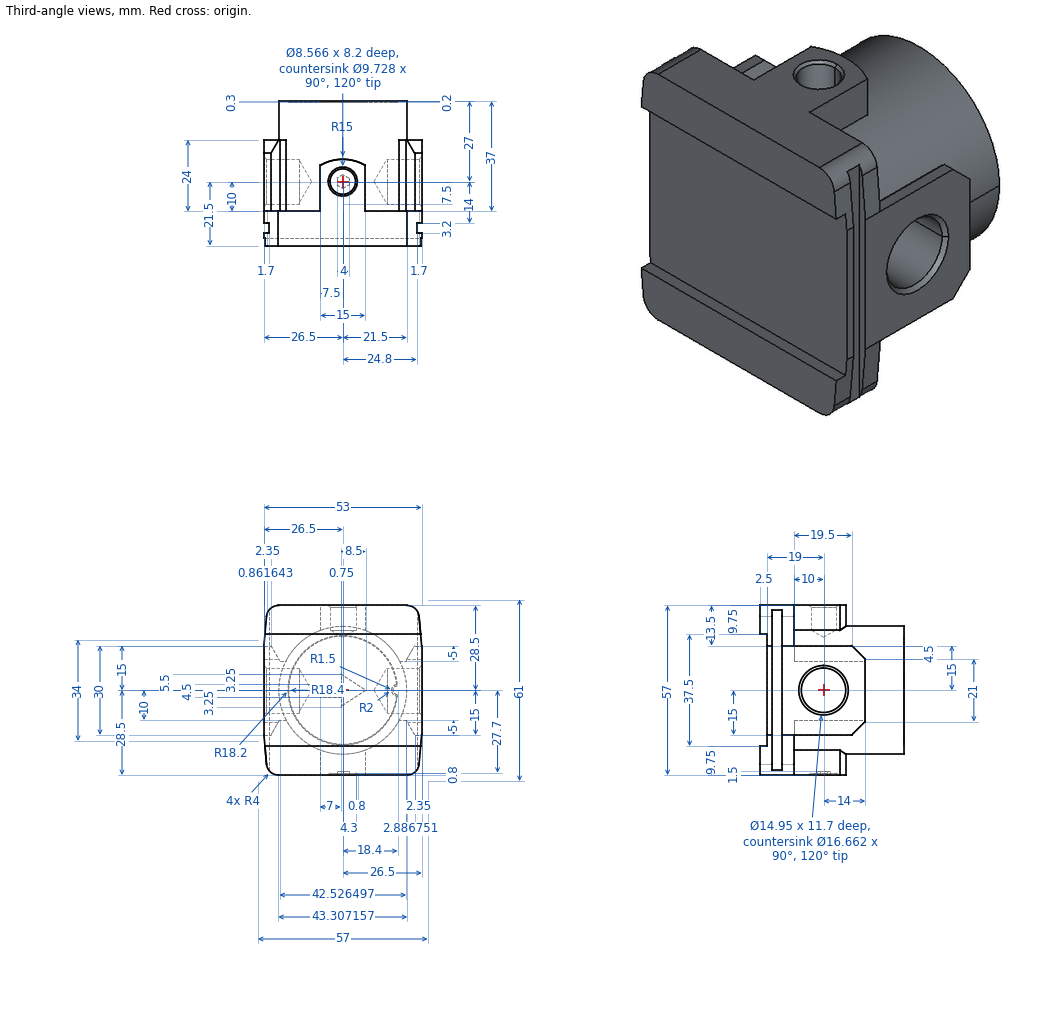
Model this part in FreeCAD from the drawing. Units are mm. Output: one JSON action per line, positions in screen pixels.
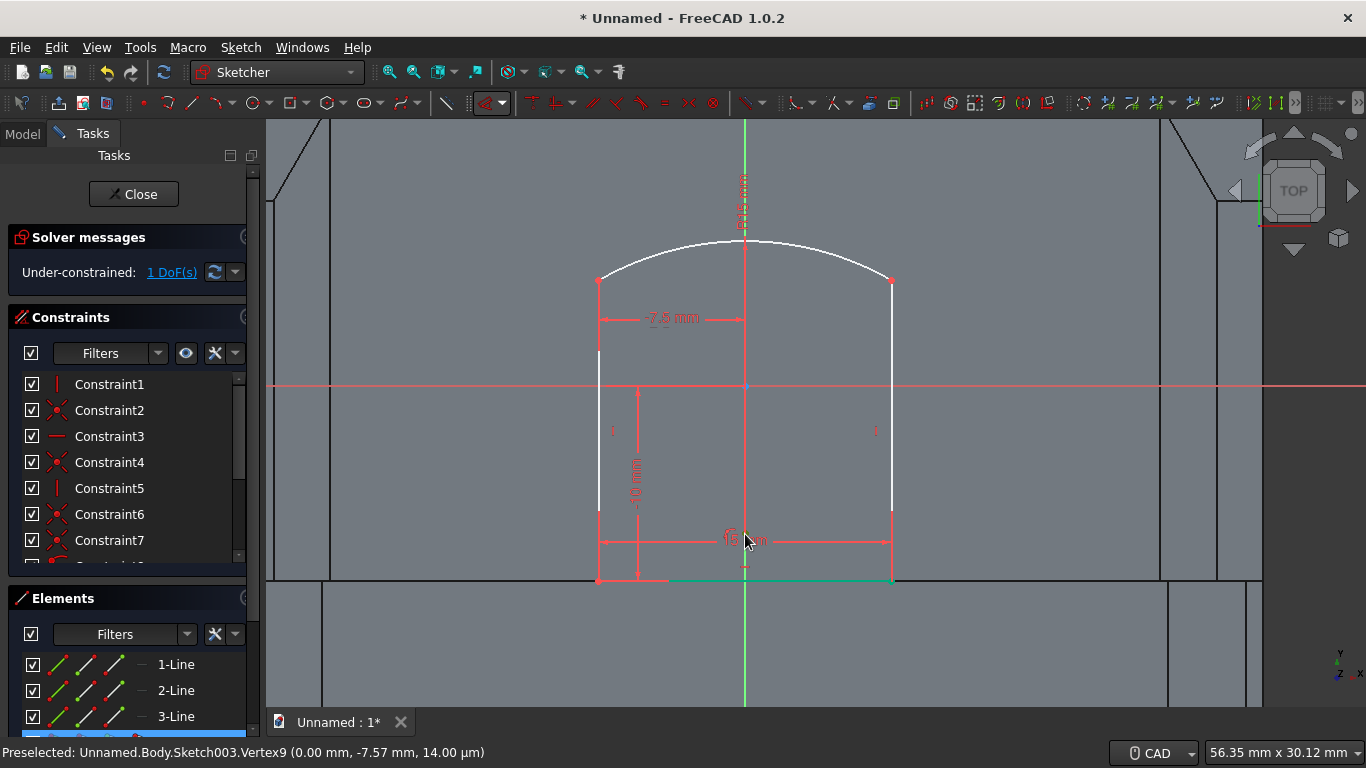
{"action": "key", "text": "i"}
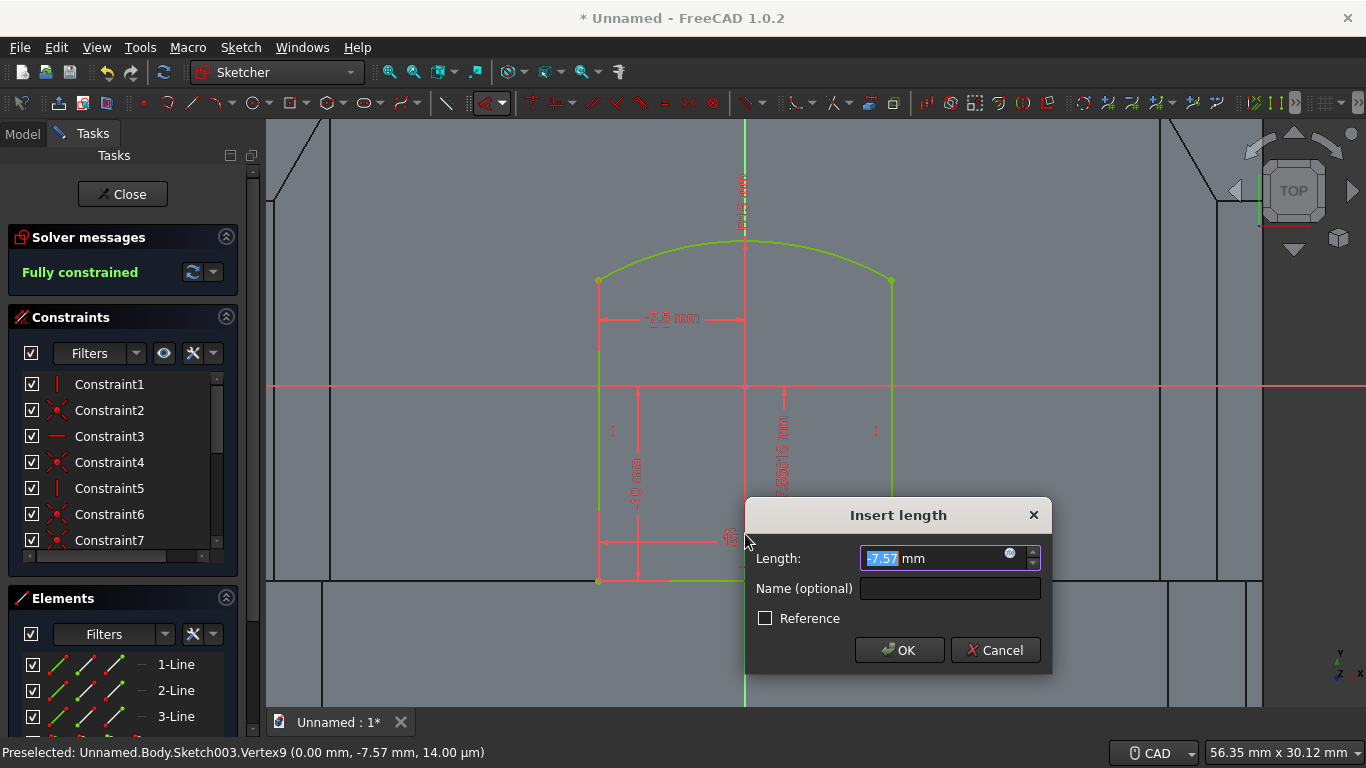
{"action": "type", "text": "-7.5"}
{"action": "key", "text": "Return"}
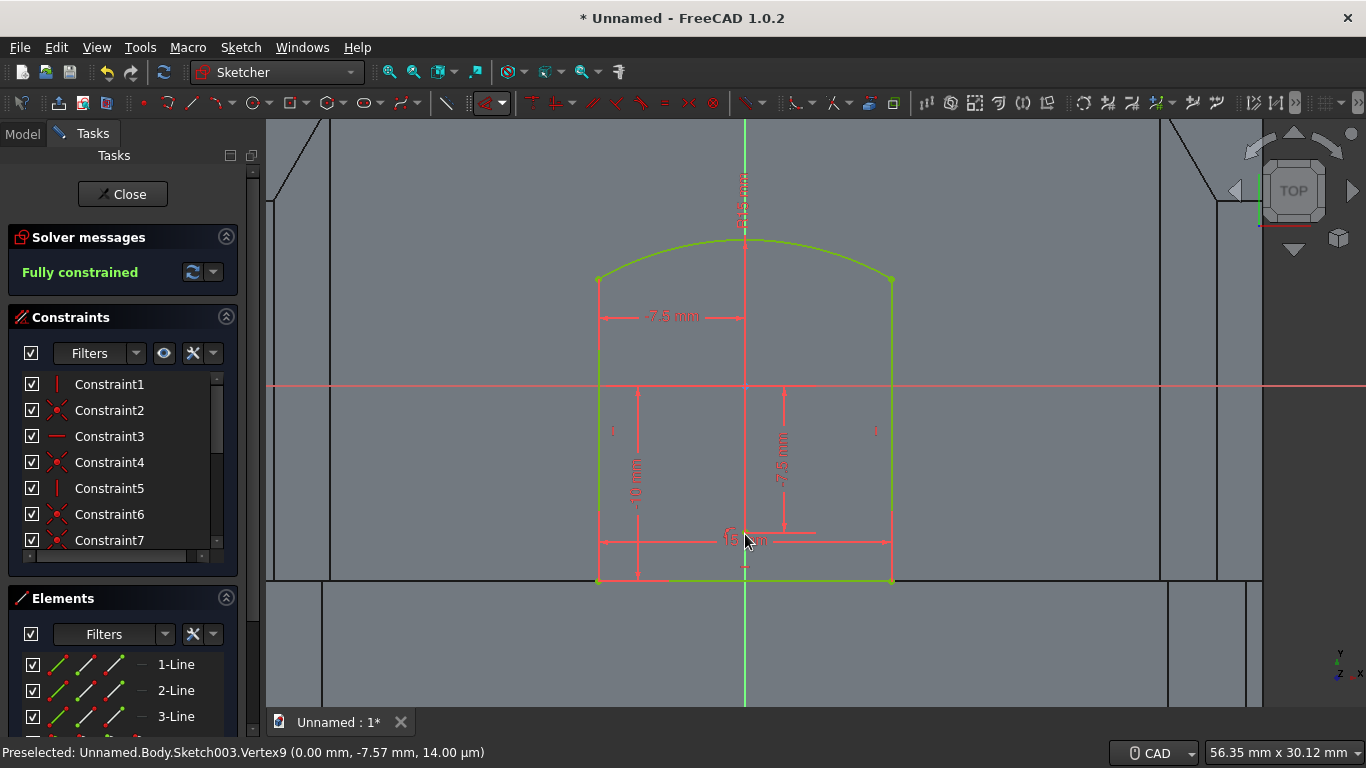
{"action": "left_click", "coordinate": [123, 194]}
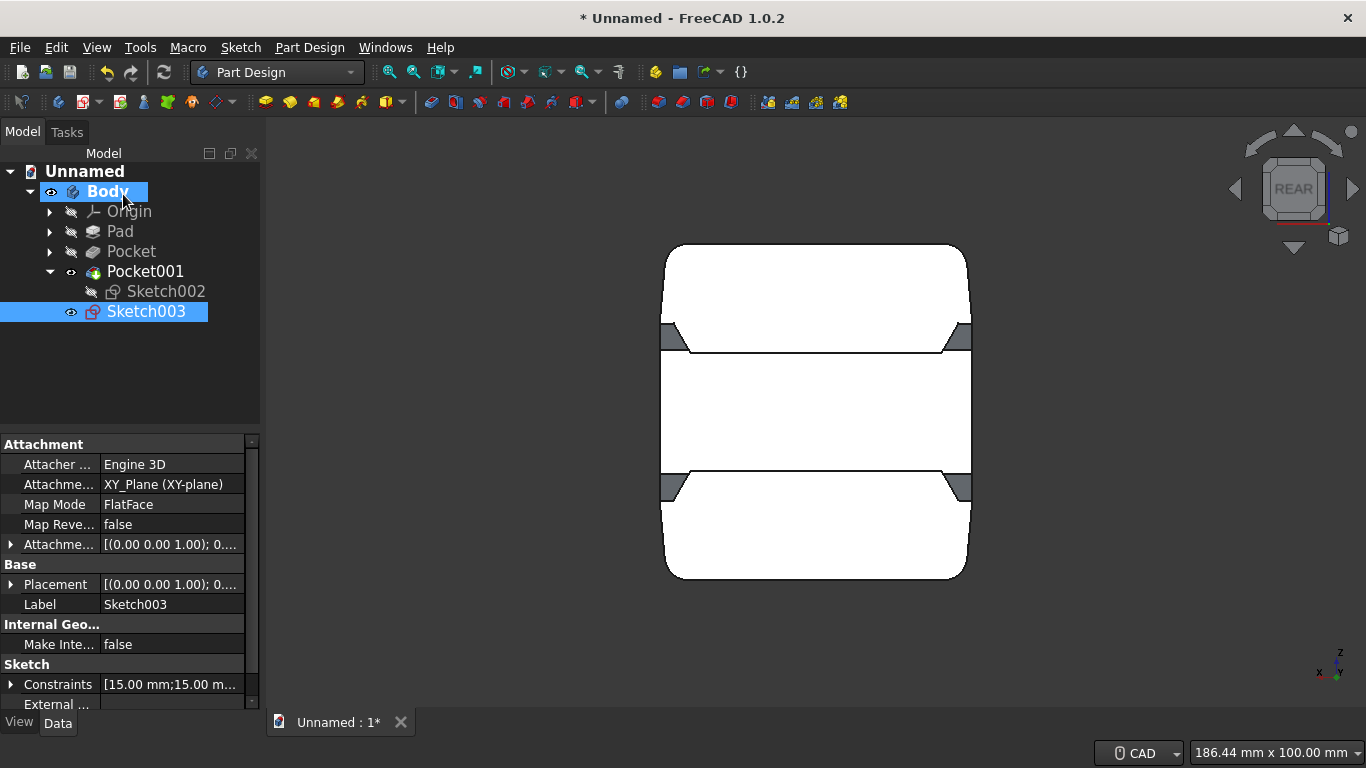
{"action": "left_click", "coordinate": [266, 102]}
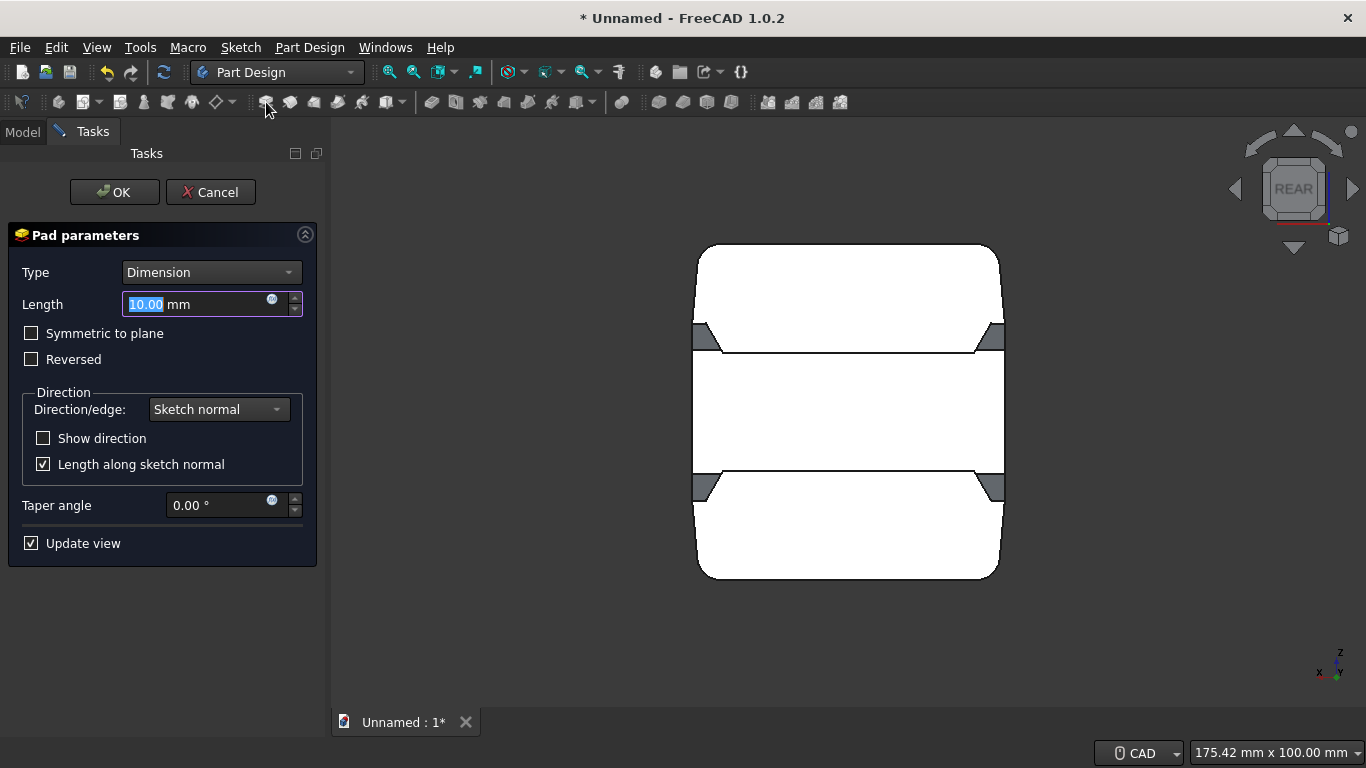
{"action": "type", "text": "57"}
{"action": "key", "text": "Tab"}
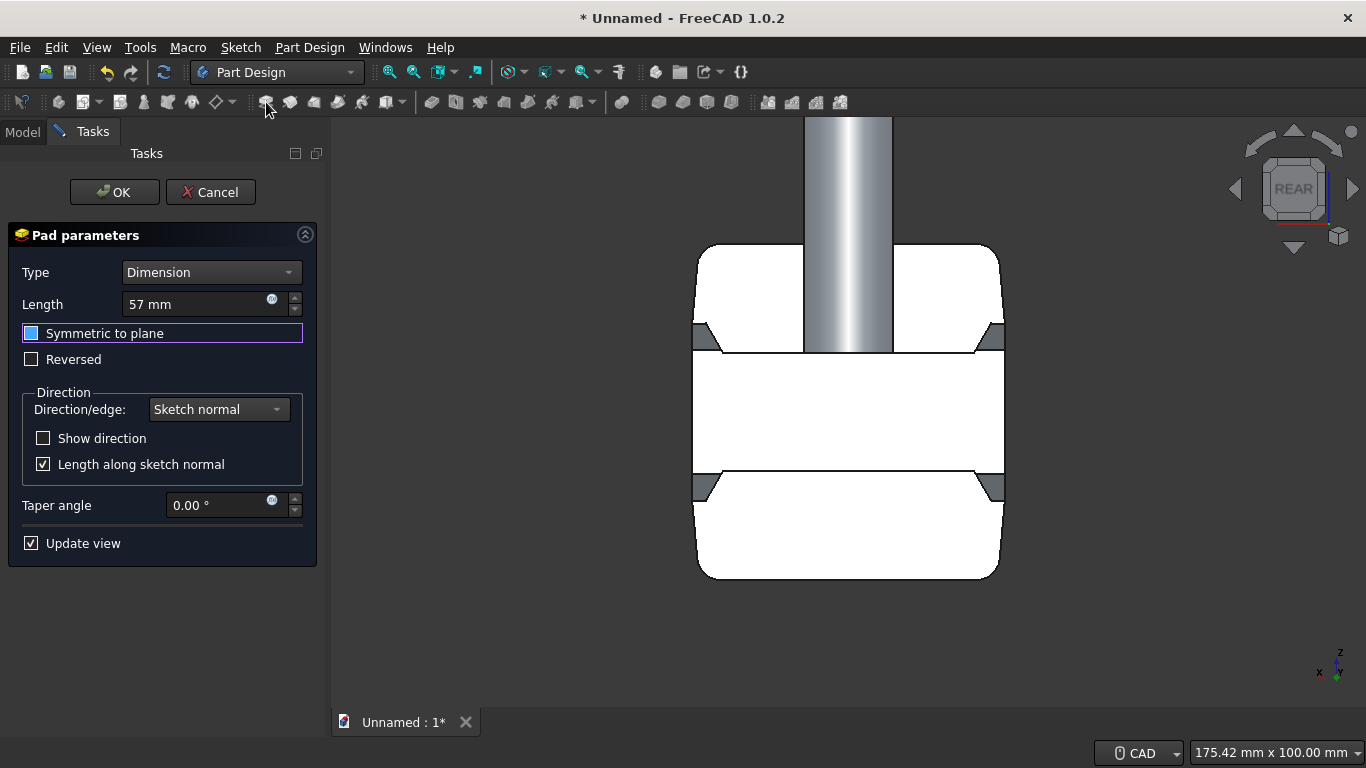
{"action": "left_click", "coordinate": [30, 333]}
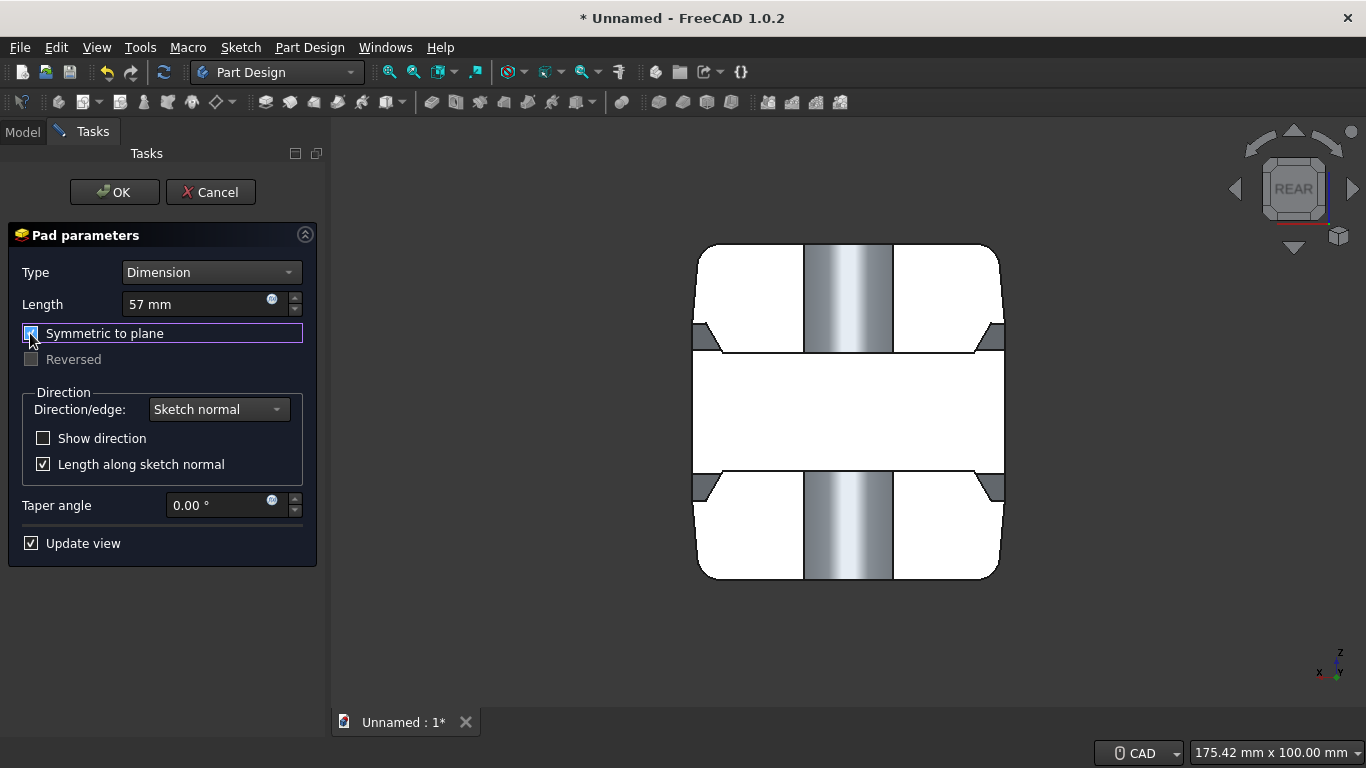
{"action": "left_click", "coordinate": [115, 192]}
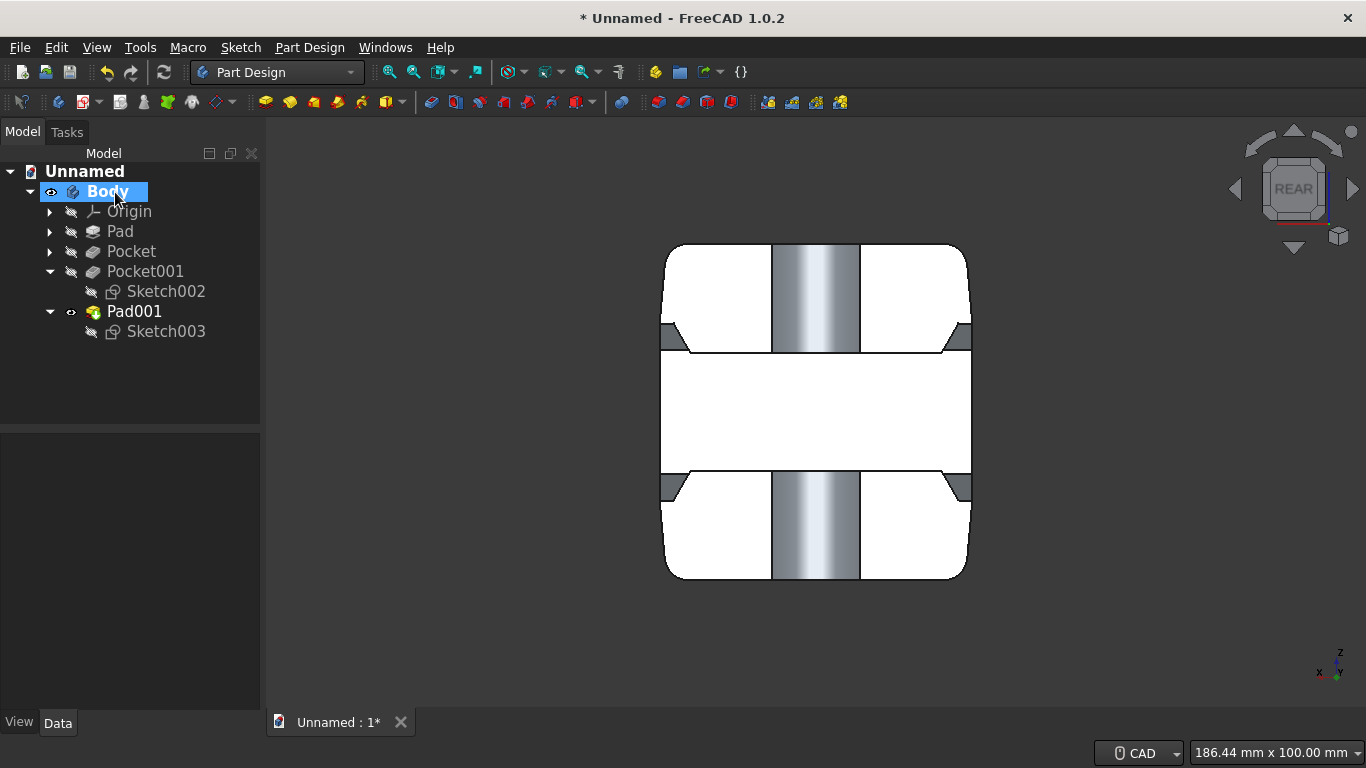
{"action": "left_click", "coordinate": [84, 102]}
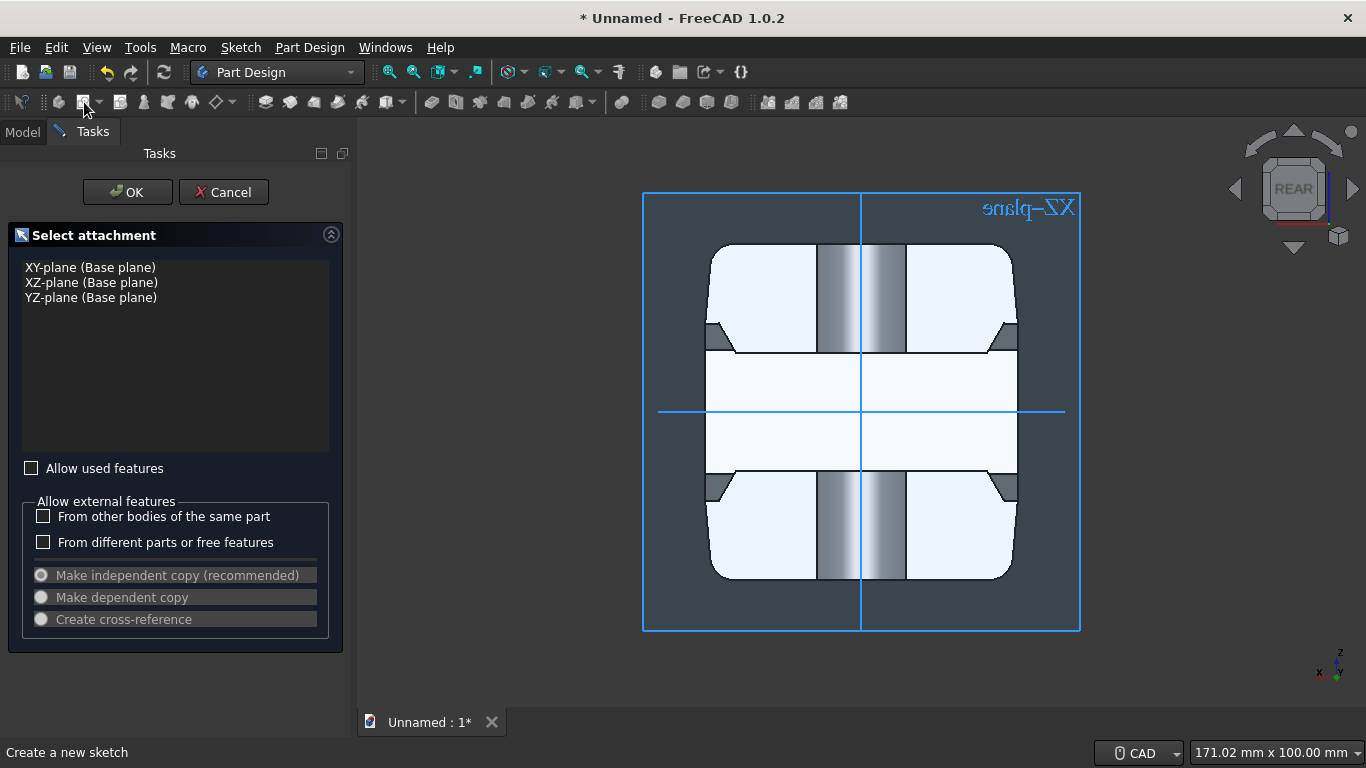
{"action": "left_click", "coordinate": [82, 268]}